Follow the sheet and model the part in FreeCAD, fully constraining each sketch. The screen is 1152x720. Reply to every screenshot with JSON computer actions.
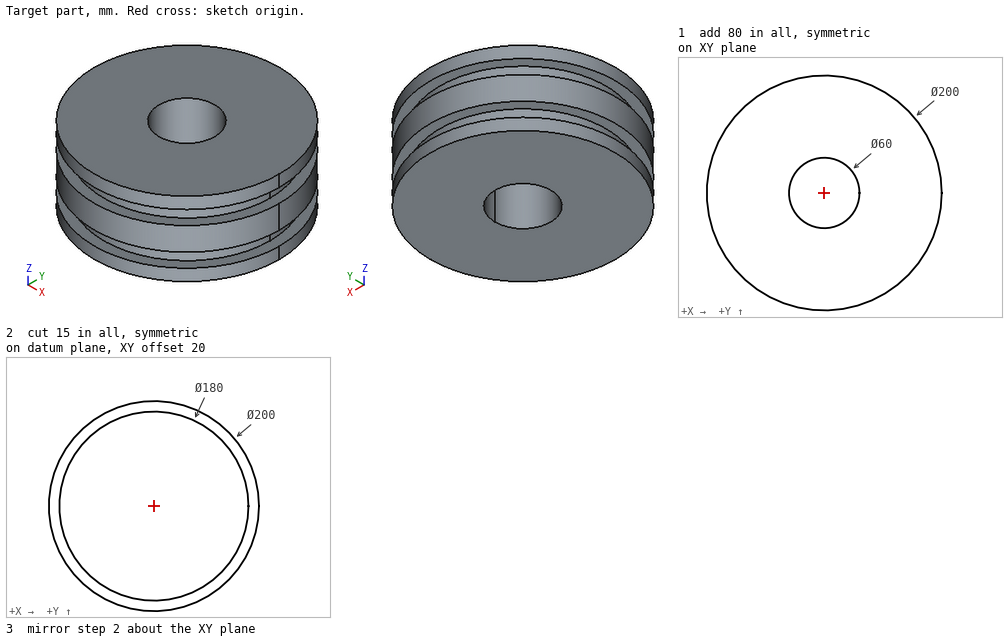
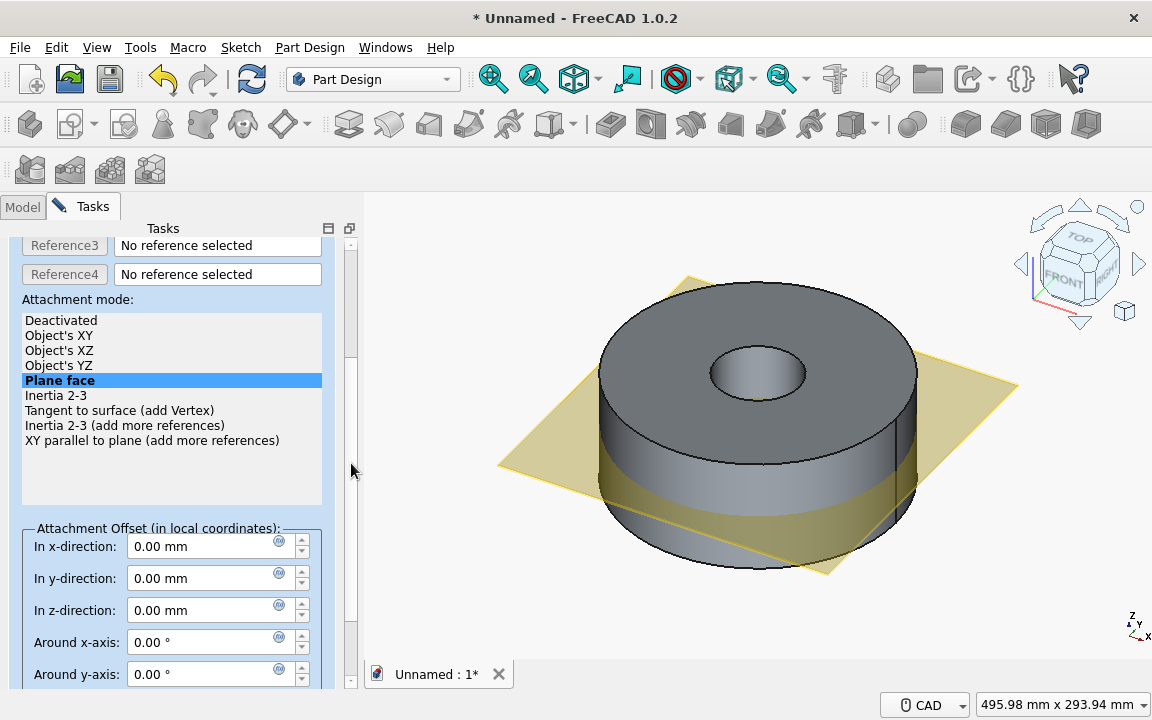
{"action": "triple_click", "coordinate": [210, 610]}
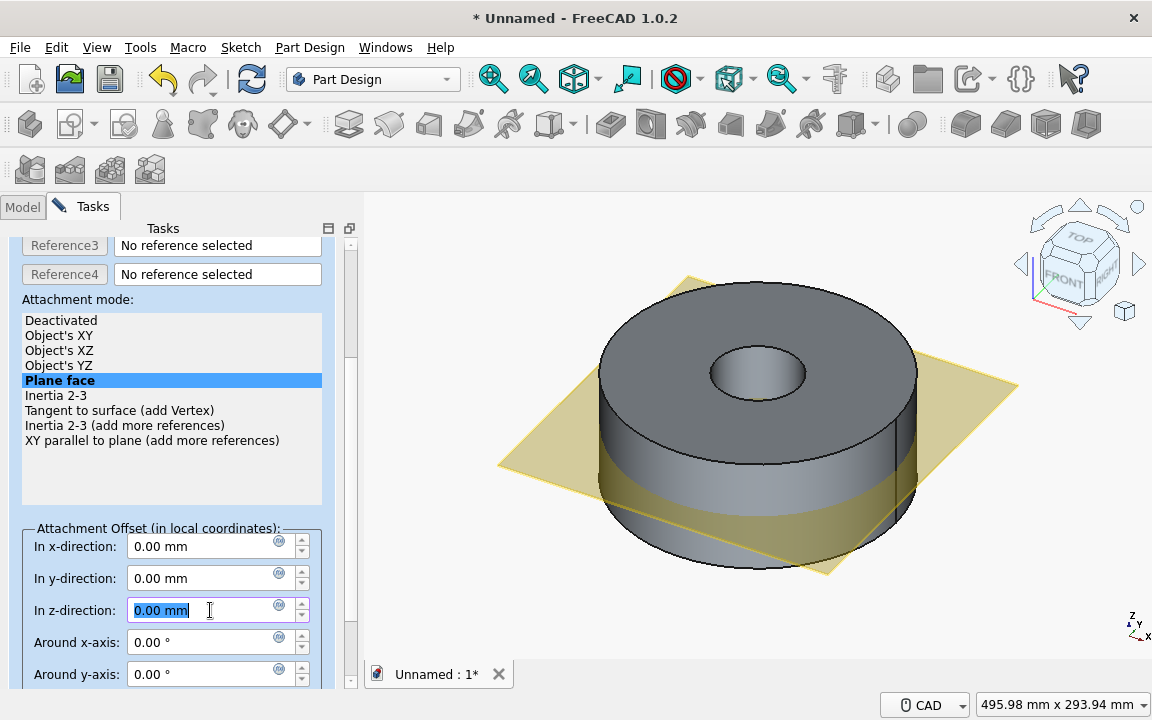
{"action": "type", "text": "20"}
{"action": "key", "text": "Tab"}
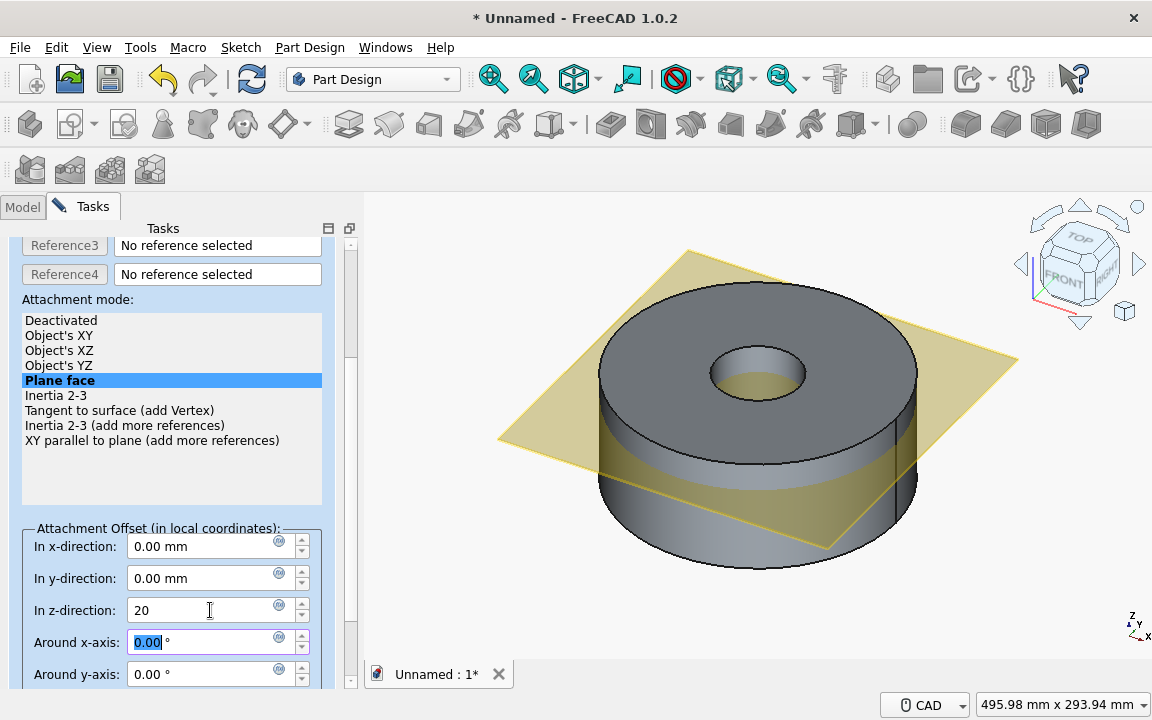
{"action": "scroll", "coordinate": [351, 463], "scroll_direction": "up", "scroll_amount": 4}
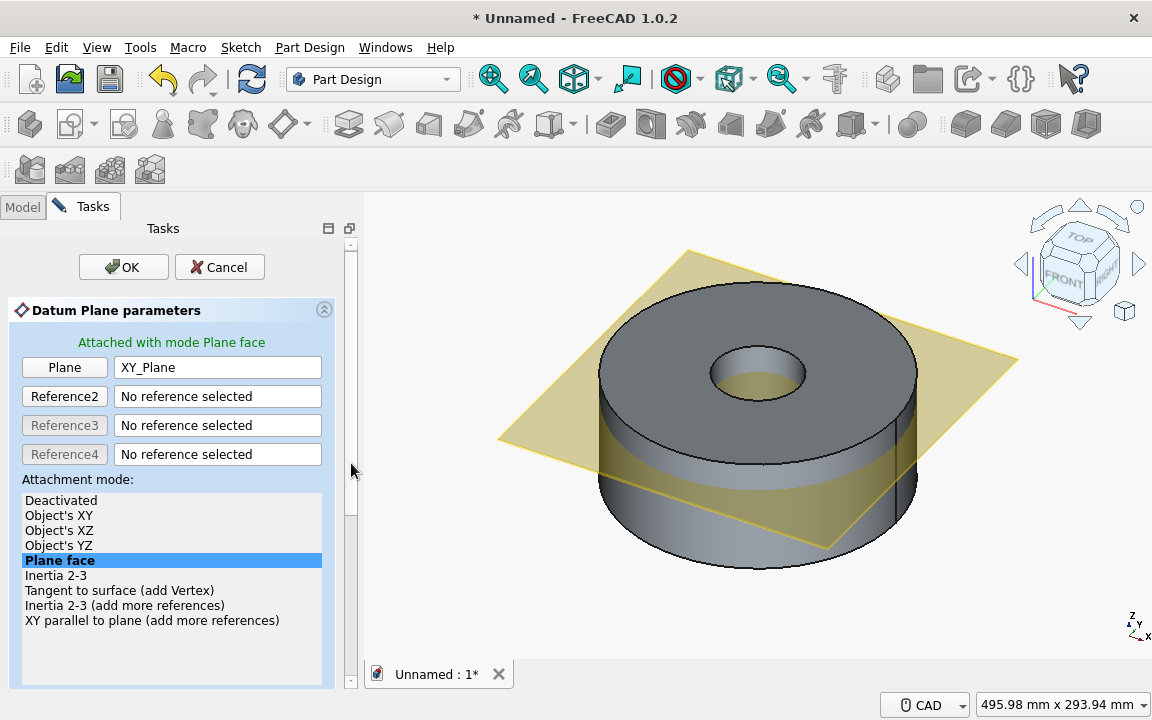
{"action": "left_click", "coordinate": [124, 267]}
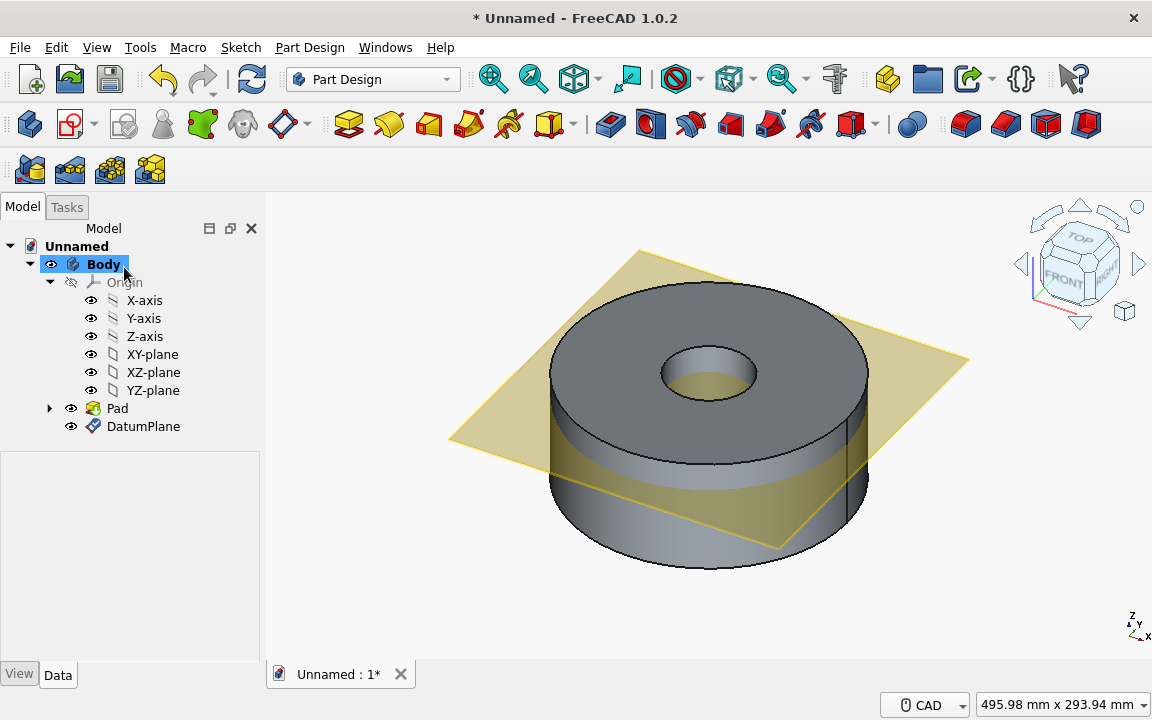
{"action": "left_click", "coordinate": [116, 426]}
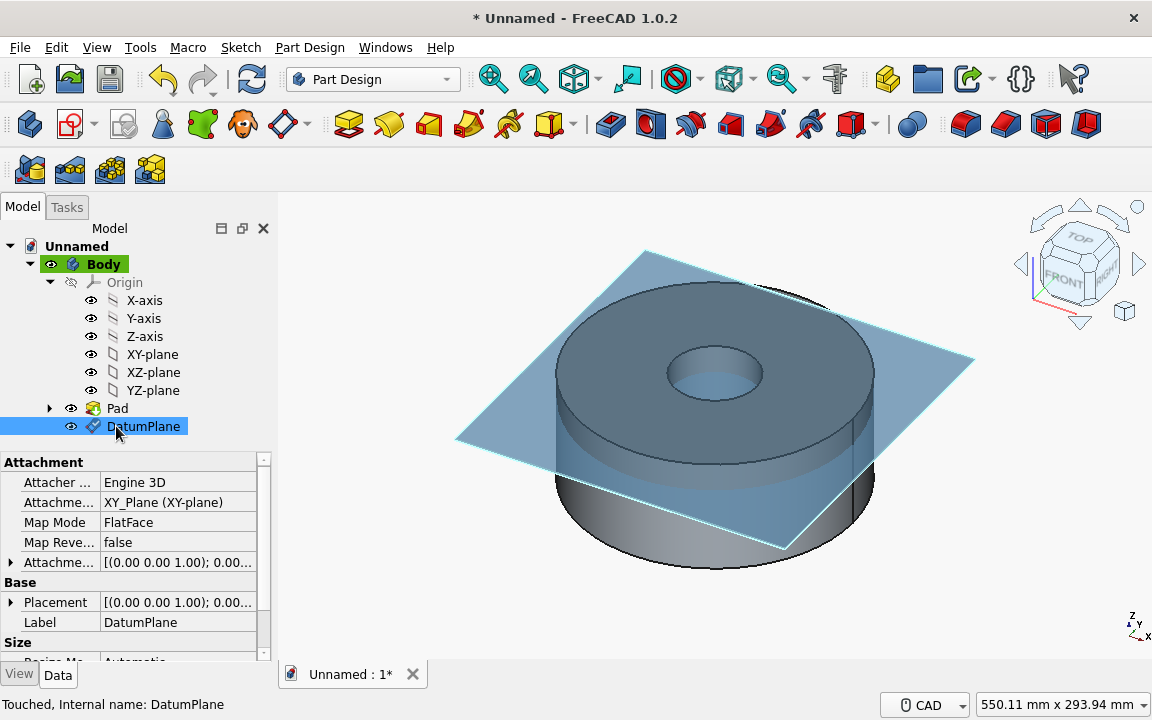
{"action": "left_click", "coordinate": [70, 124]}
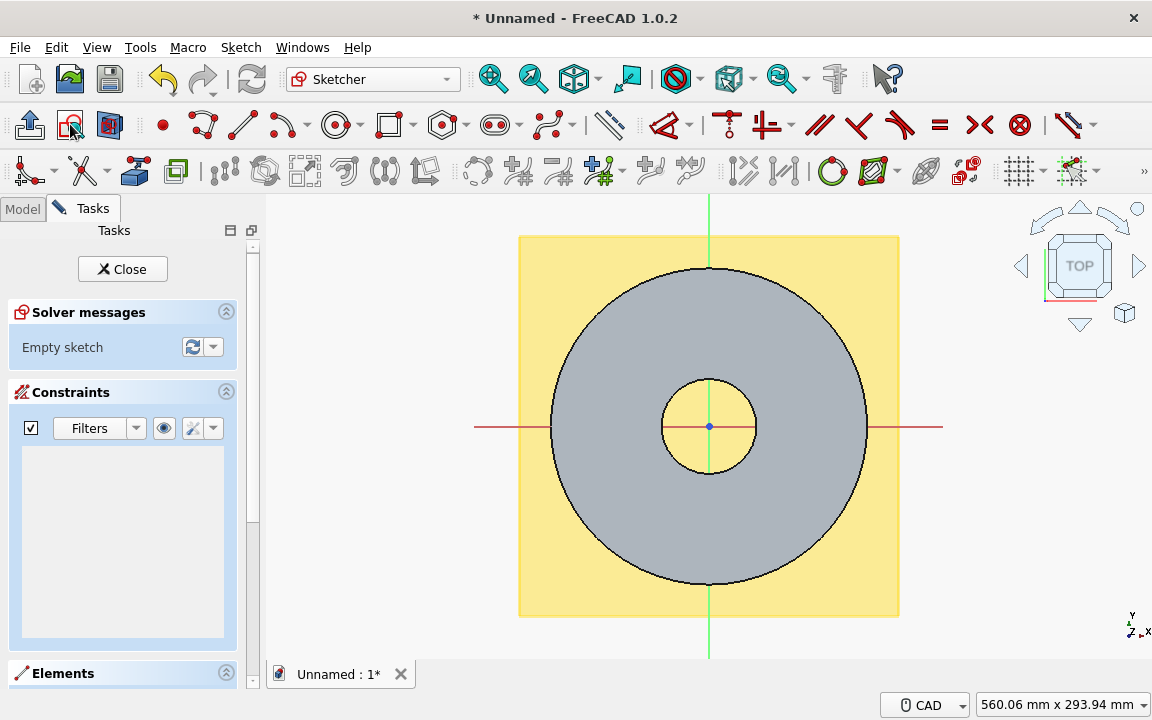
{"action": "left_click", "coordinate": [110, 126]}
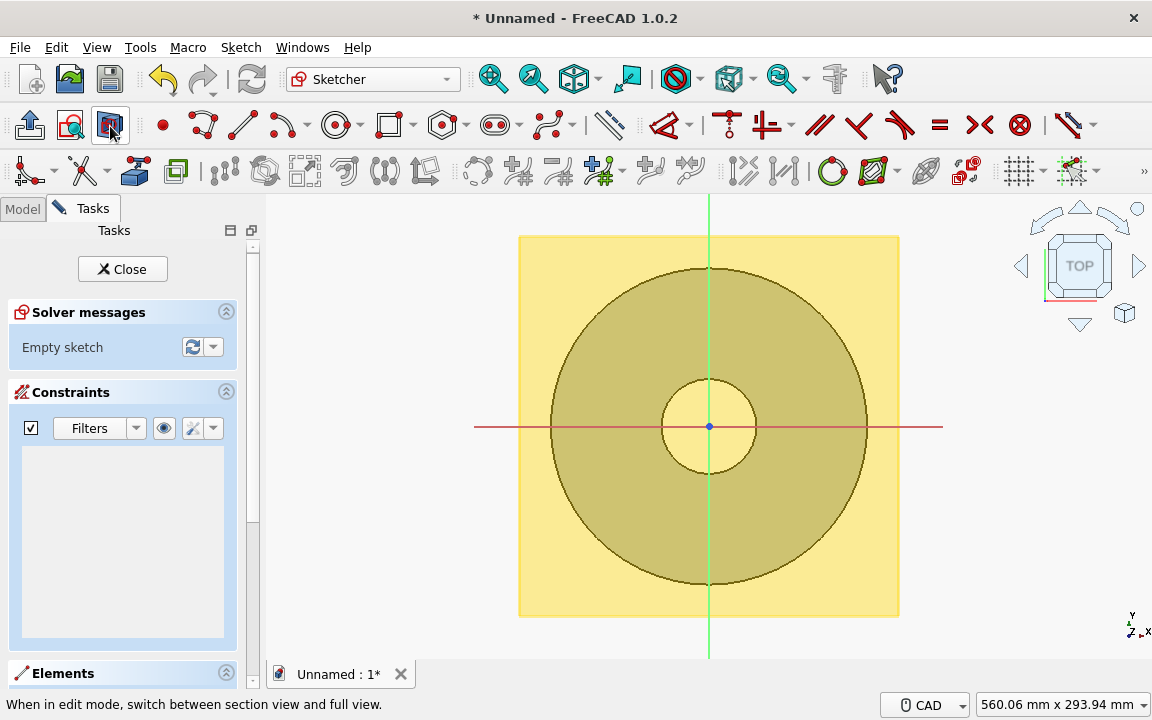
{"action": "left_click", "coordinate": [336, 126]}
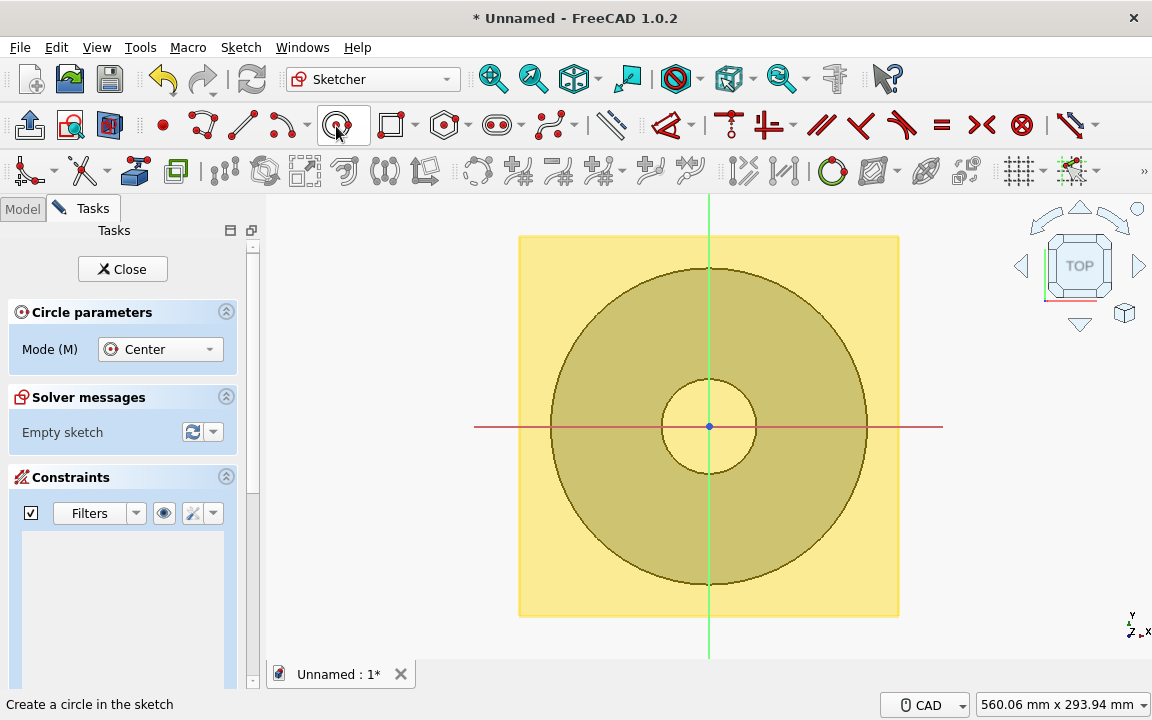
{"action": "left_click", "coordinate": [709, 426]}
{"action": "left_click", "coordinate": [821, 315]}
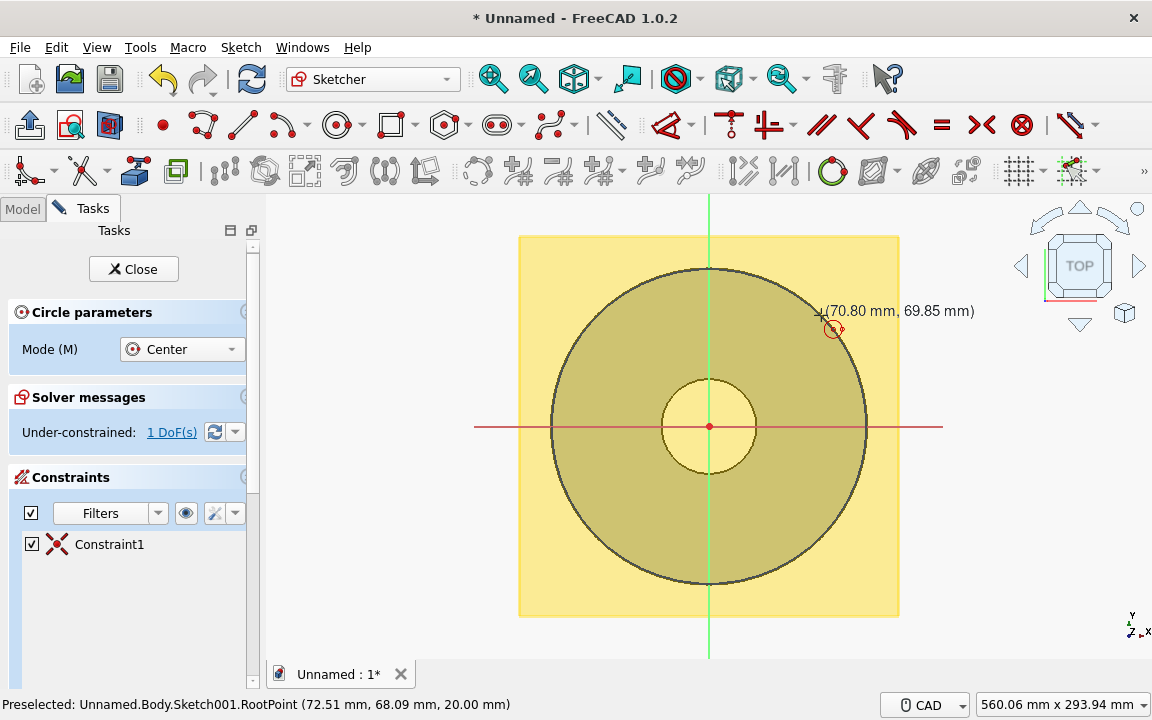
{"action": "left_click", "coordinate": [709, 426]}
{"action": "left_click", "coordinate": [810, 326]}
{"action": "key", "text": "Escape"}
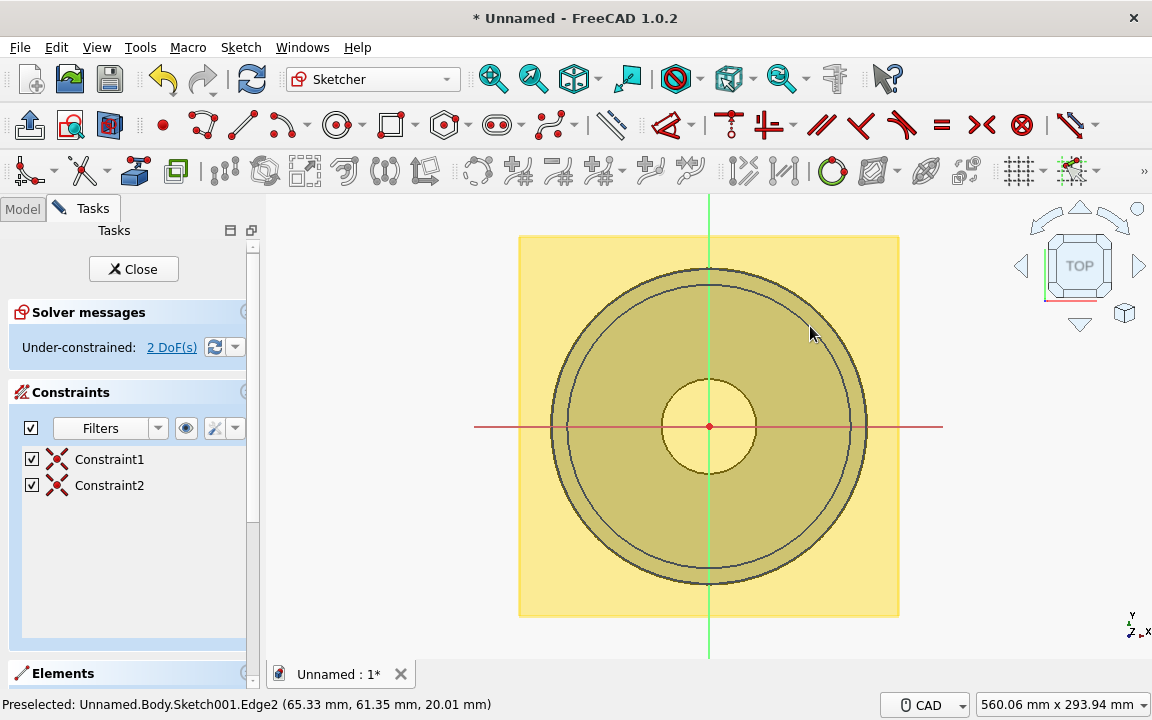
{"action": "left_click", "coordinate": [666, 126]}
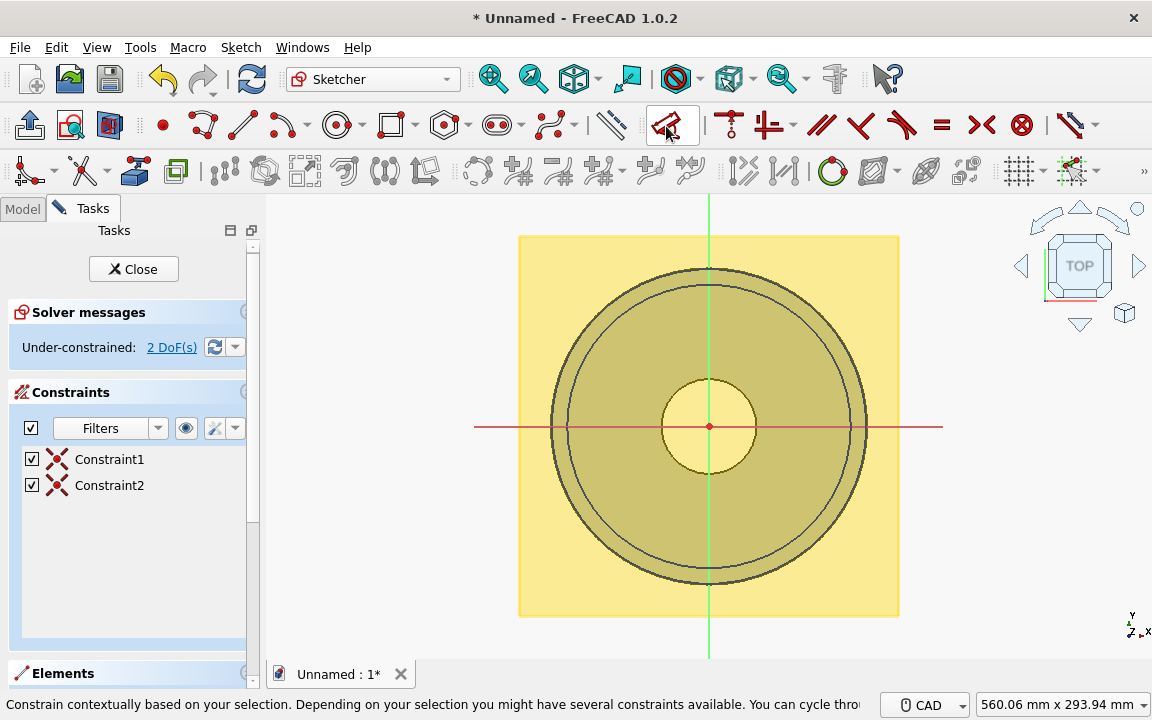
{"action": "left_click", "coordinate": [820, 315]}
{"action": "left_click", "coordinate": [843, 292]}